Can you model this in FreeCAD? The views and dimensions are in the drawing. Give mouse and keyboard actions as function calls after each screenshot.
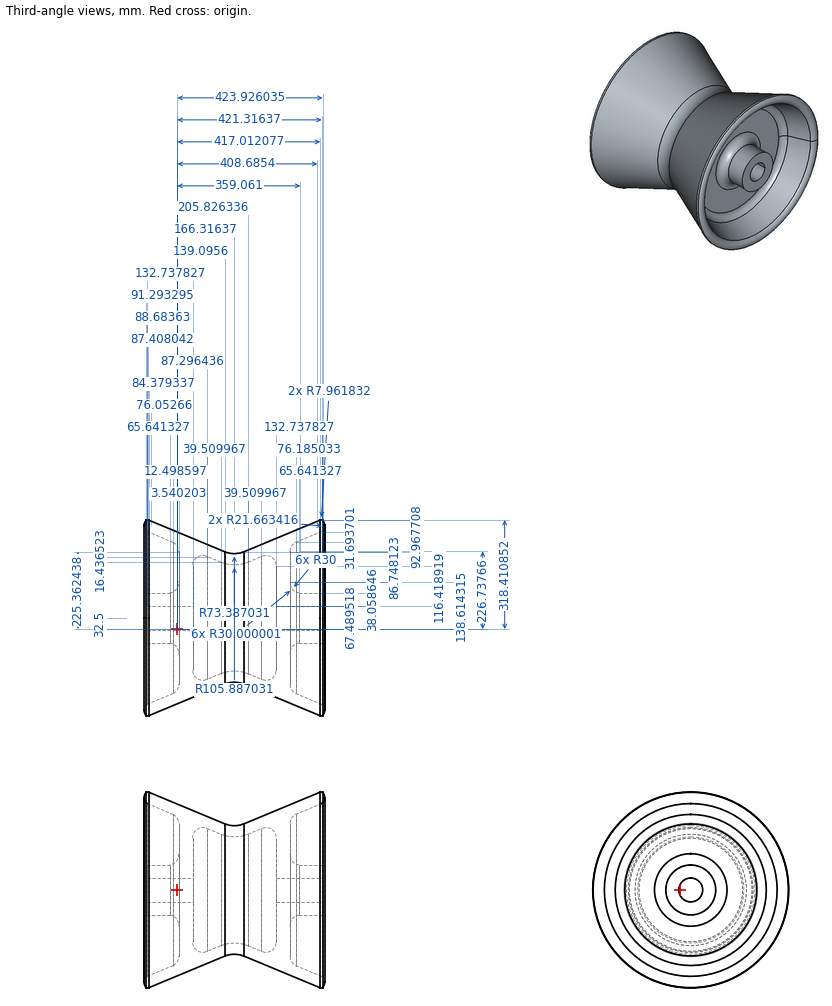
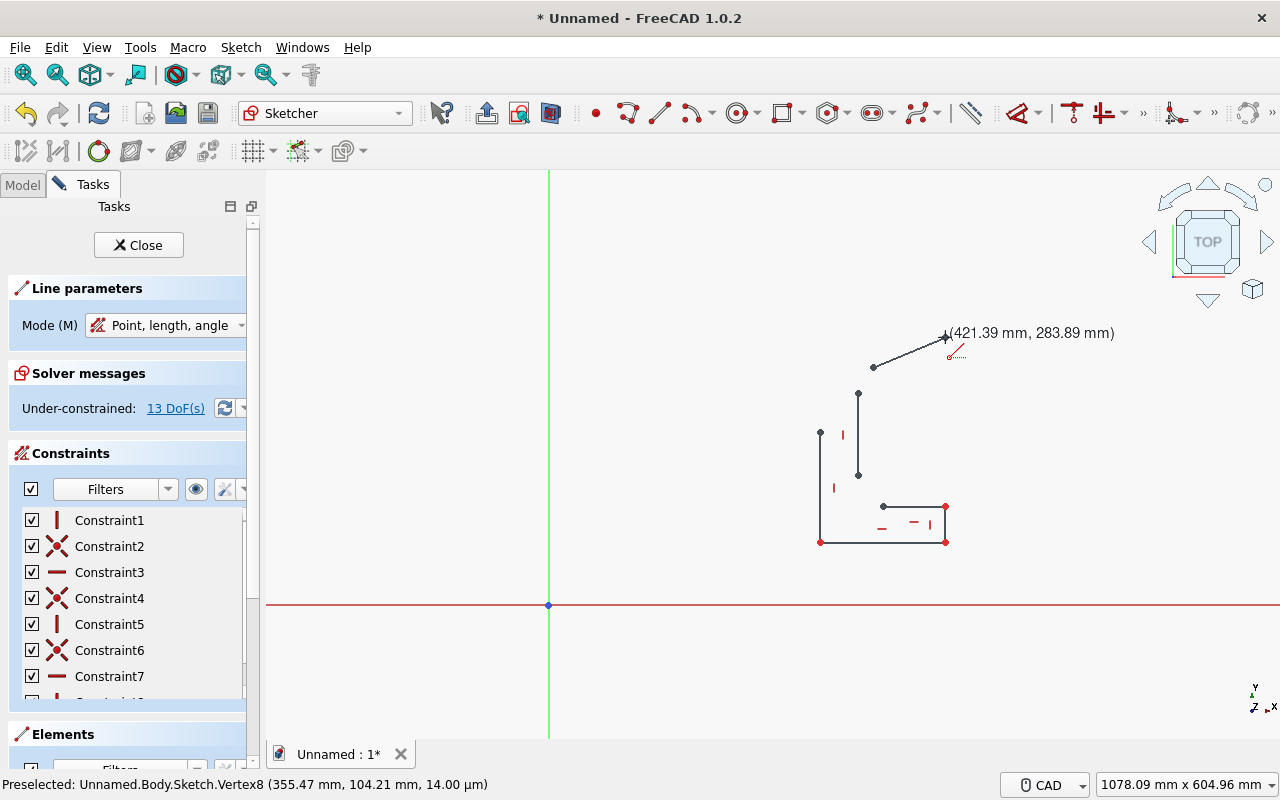
click(941, 306)
click(731, 393)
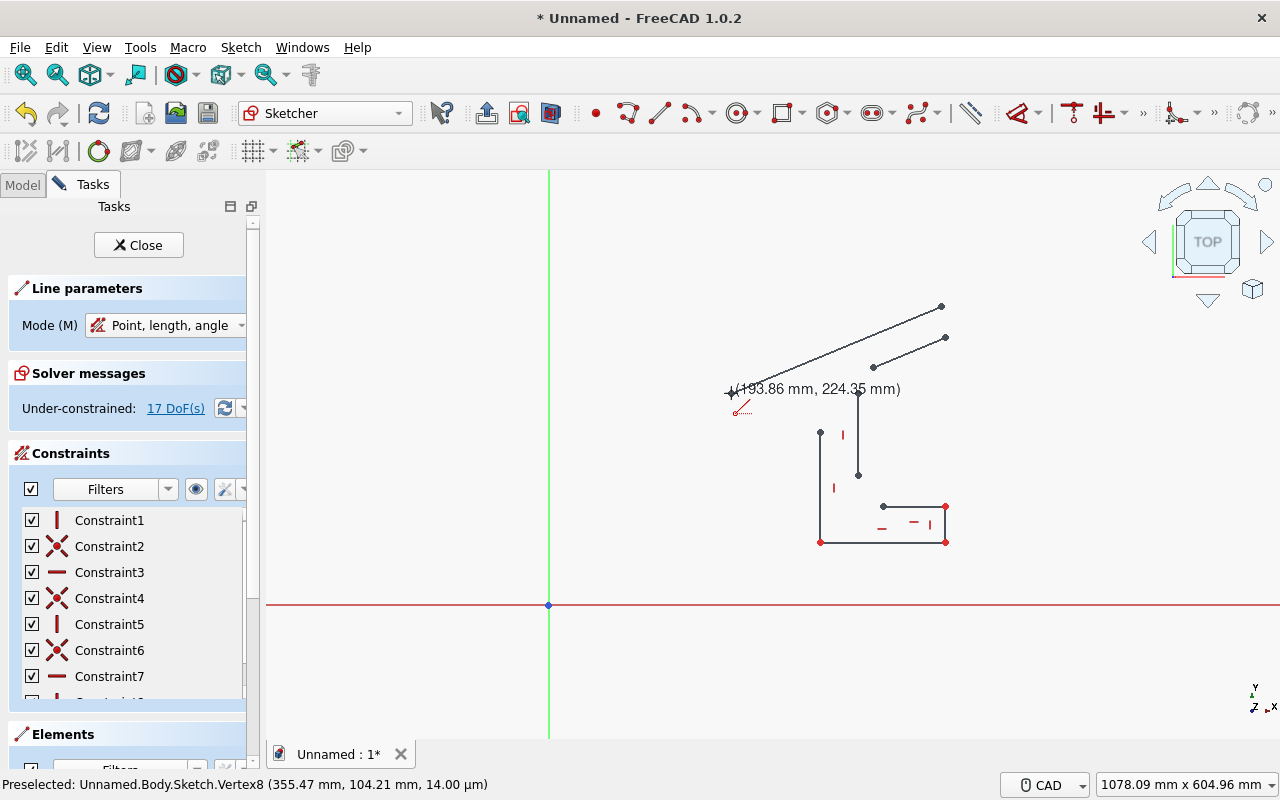
click(679, 393)
click(469, 306)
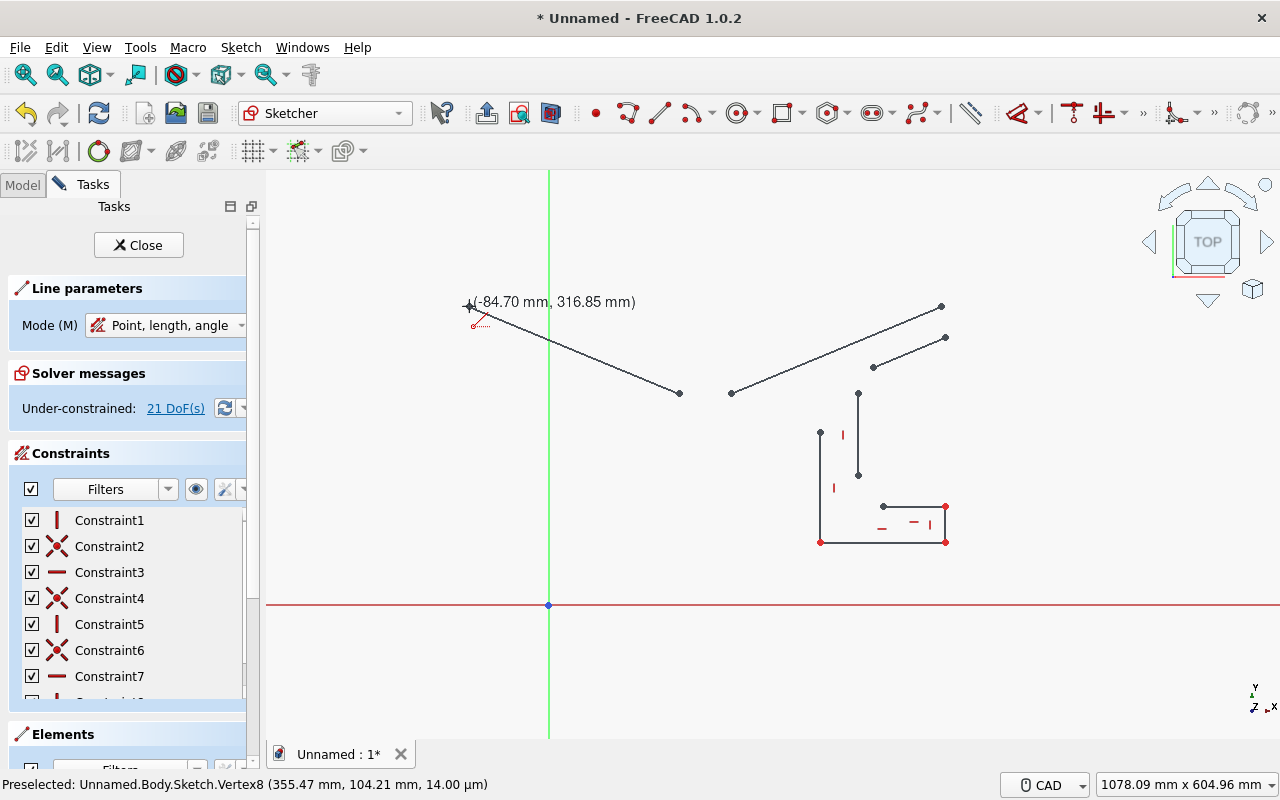
click(465, 337)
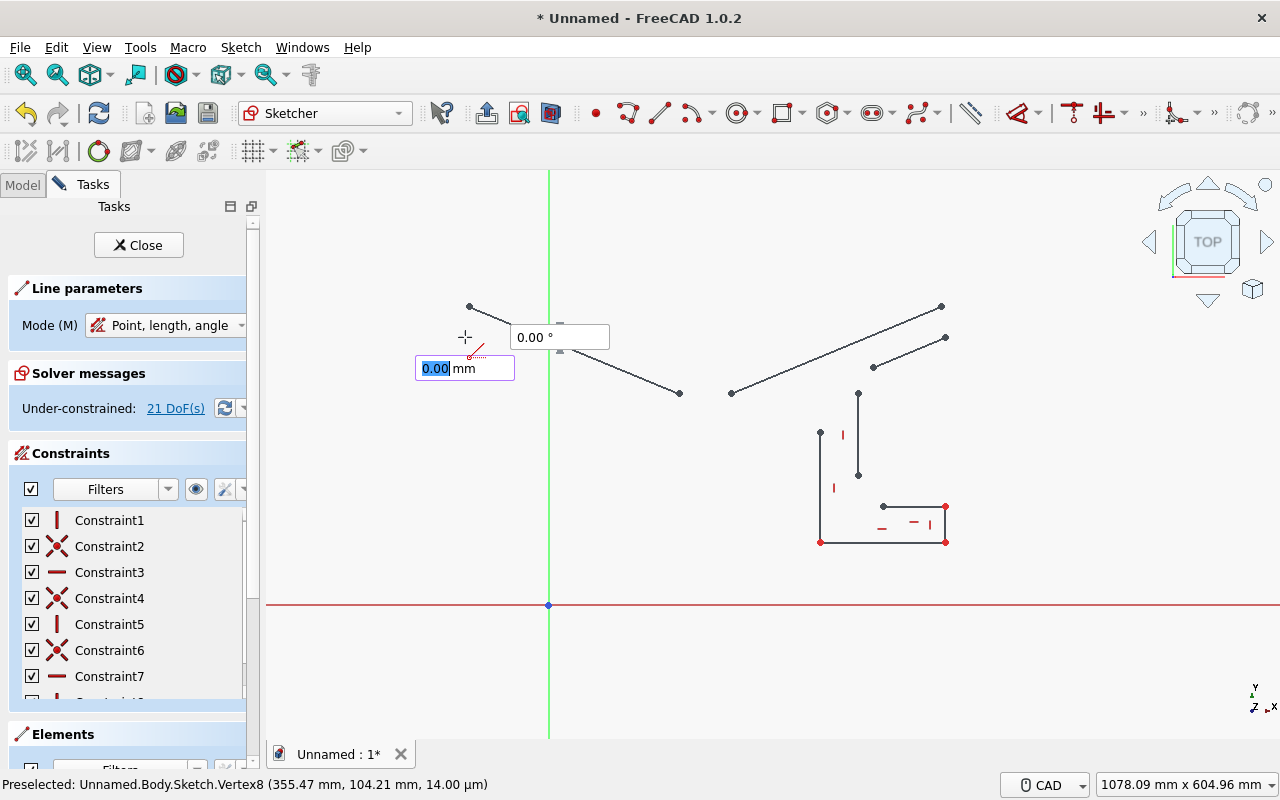
scroll(537, 367, up, 2)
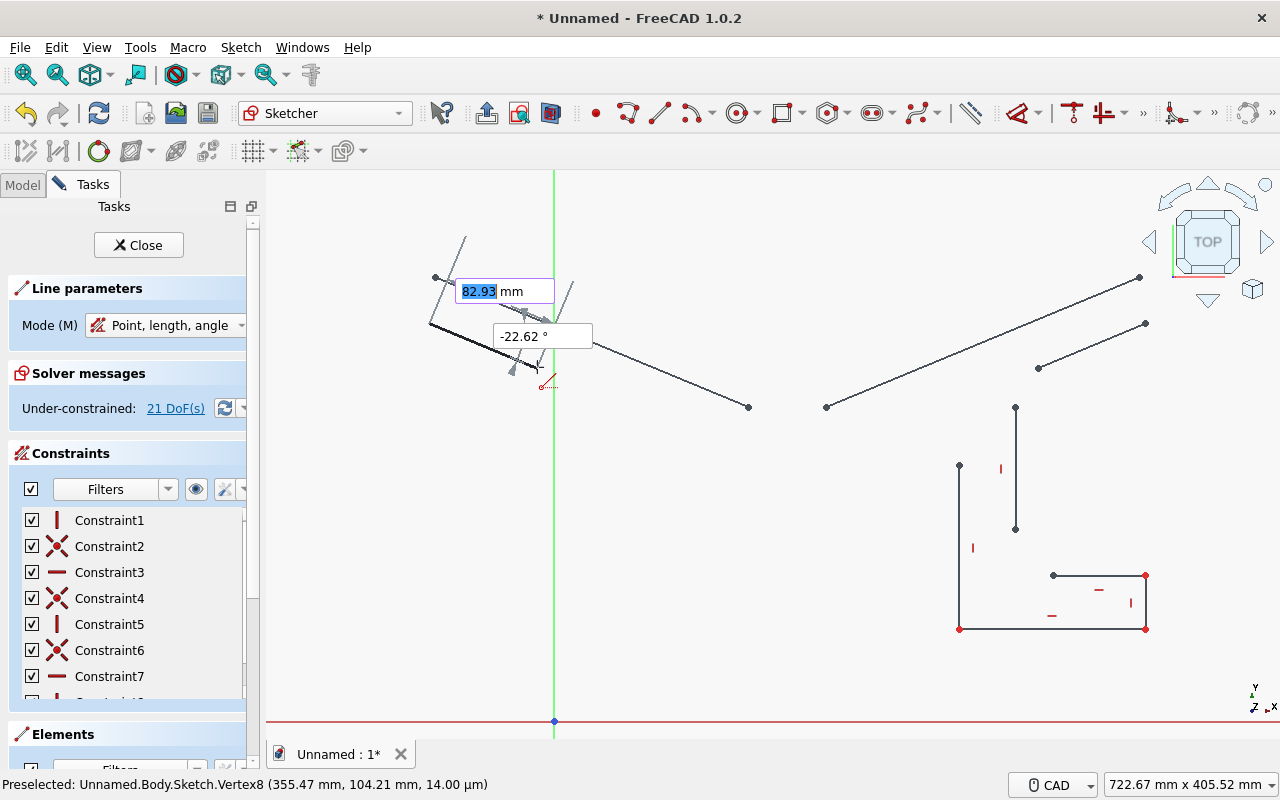
click(537, 366)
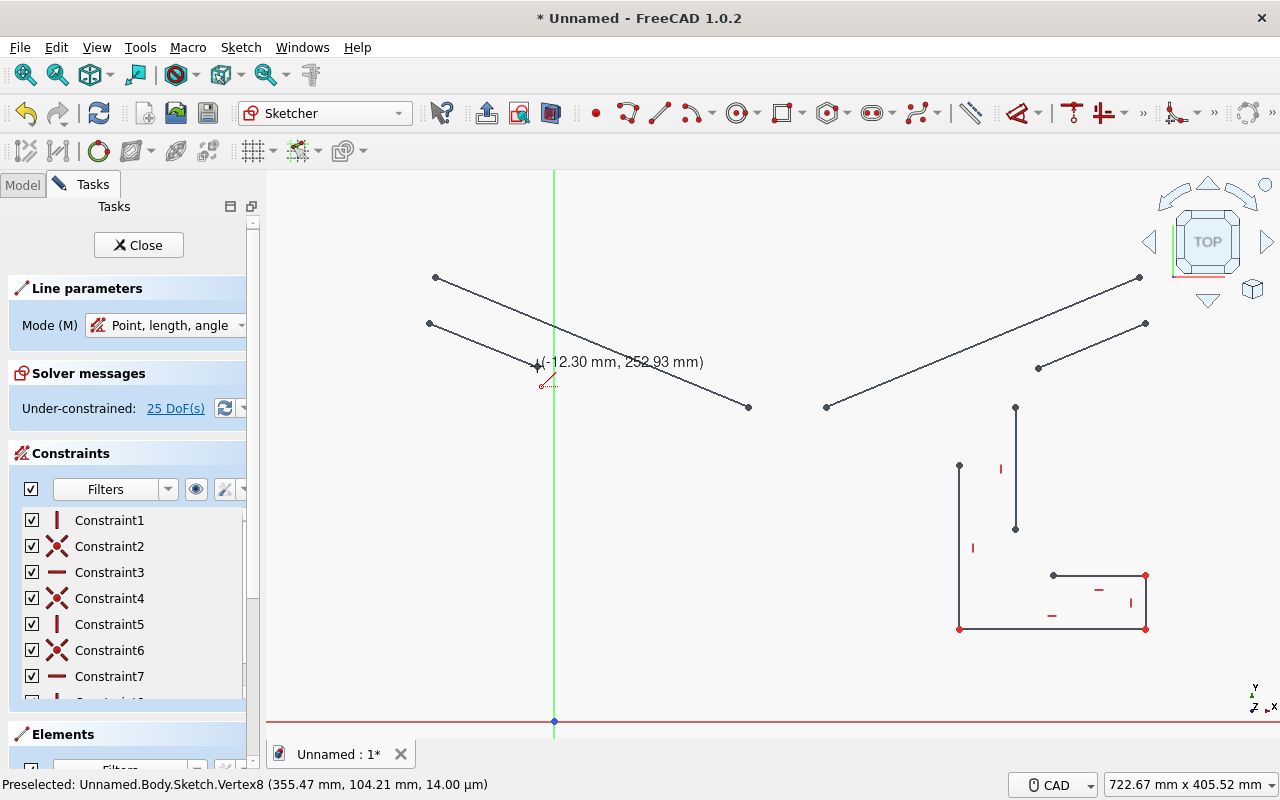
scroll(559, 406, up, 6)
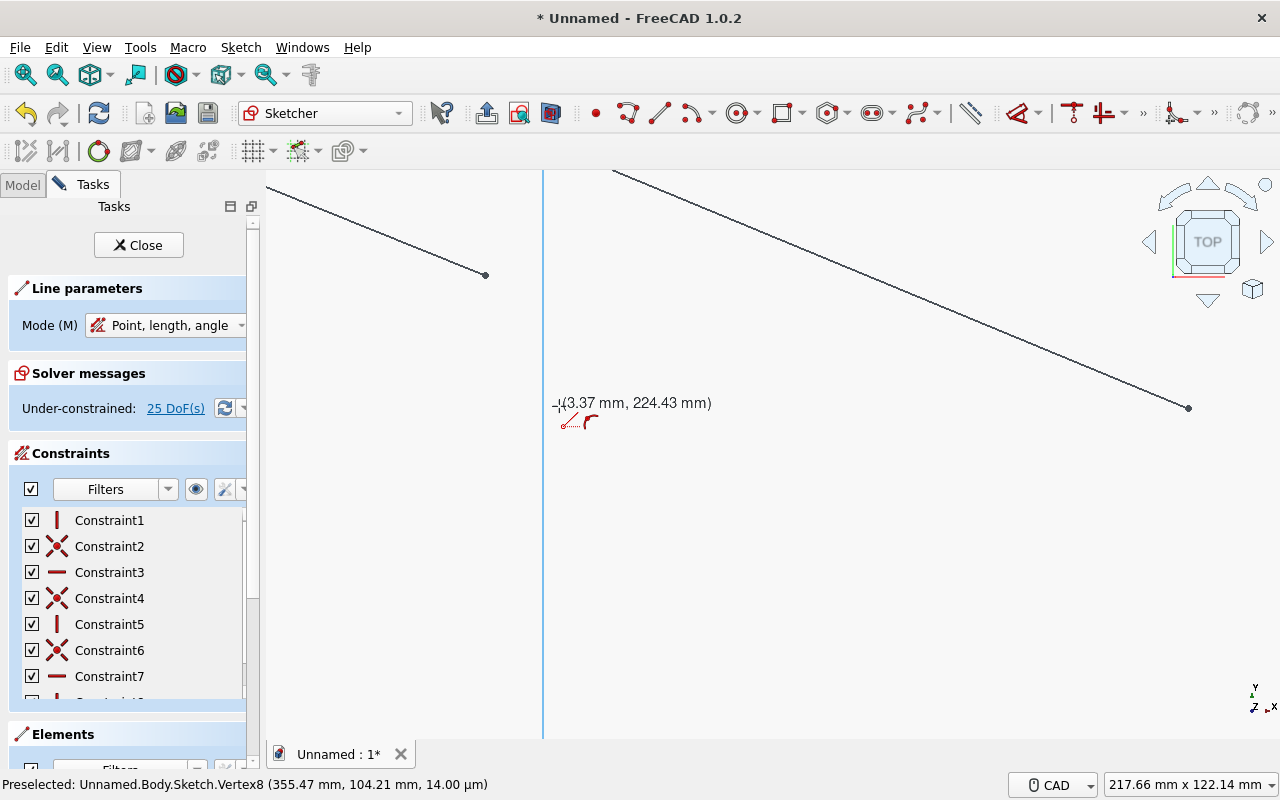
click(559, 404)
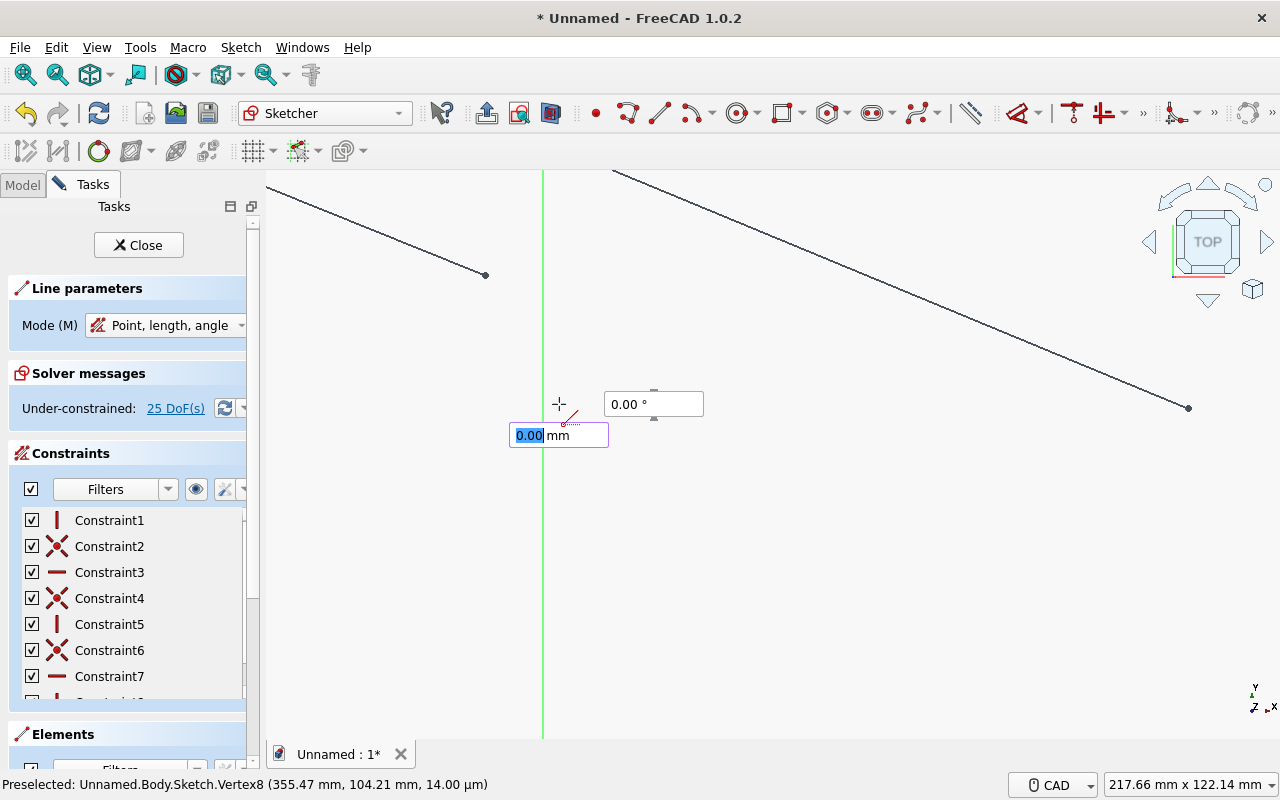
scroll(549, 390, down, 8)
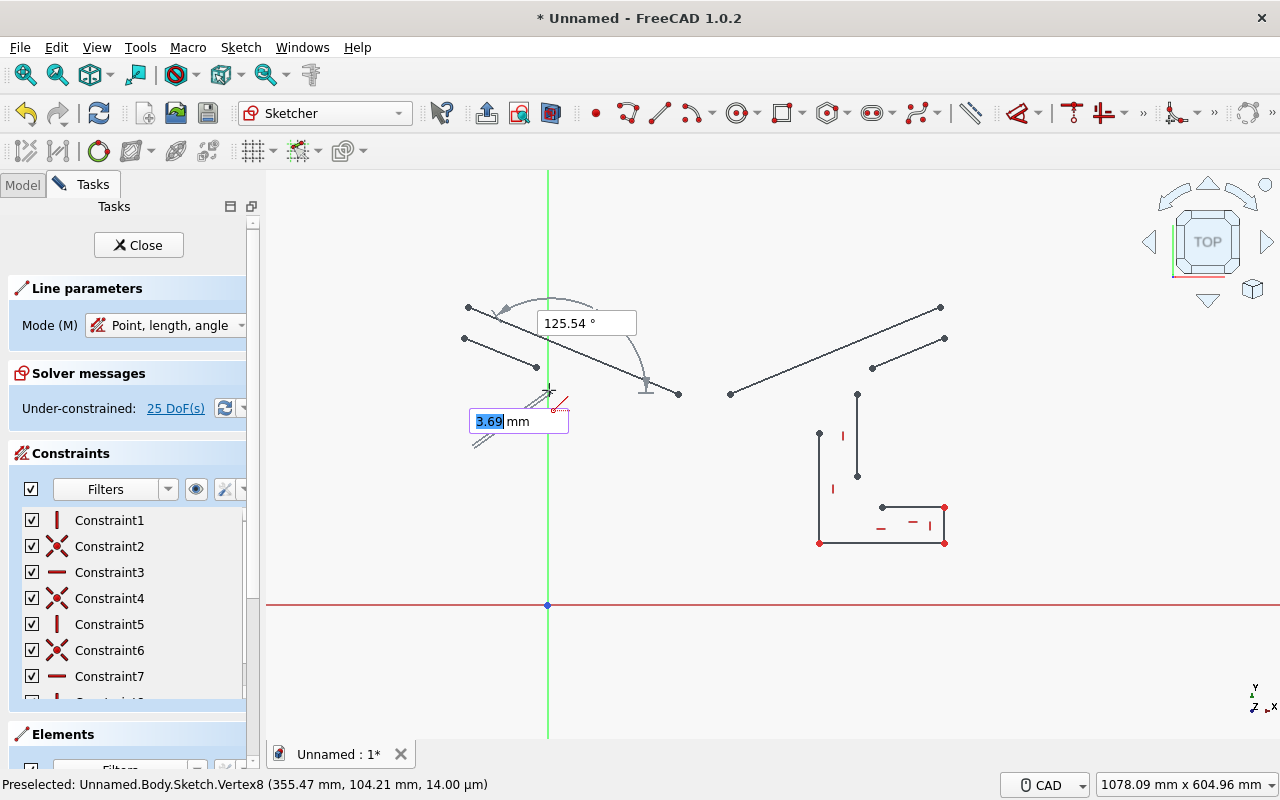
scroll(551, 475, up, 8)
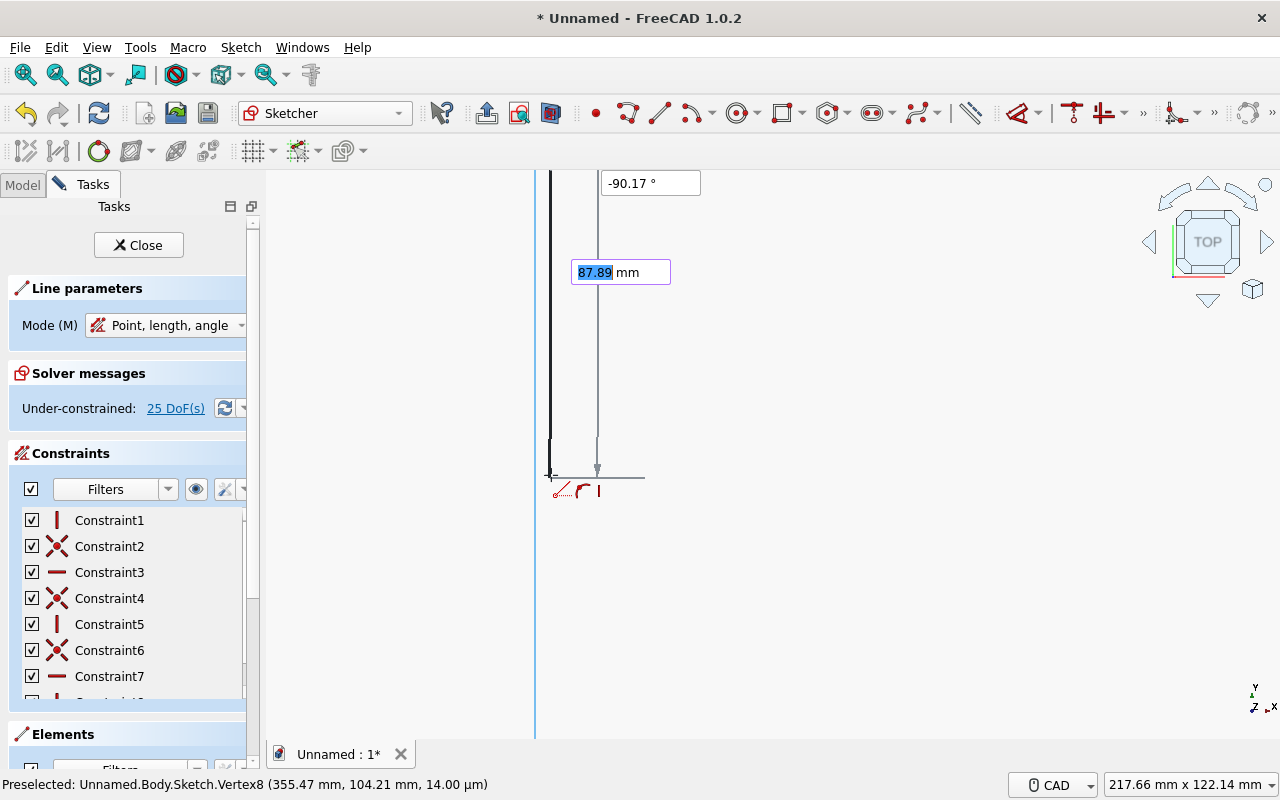
click(551, 472)